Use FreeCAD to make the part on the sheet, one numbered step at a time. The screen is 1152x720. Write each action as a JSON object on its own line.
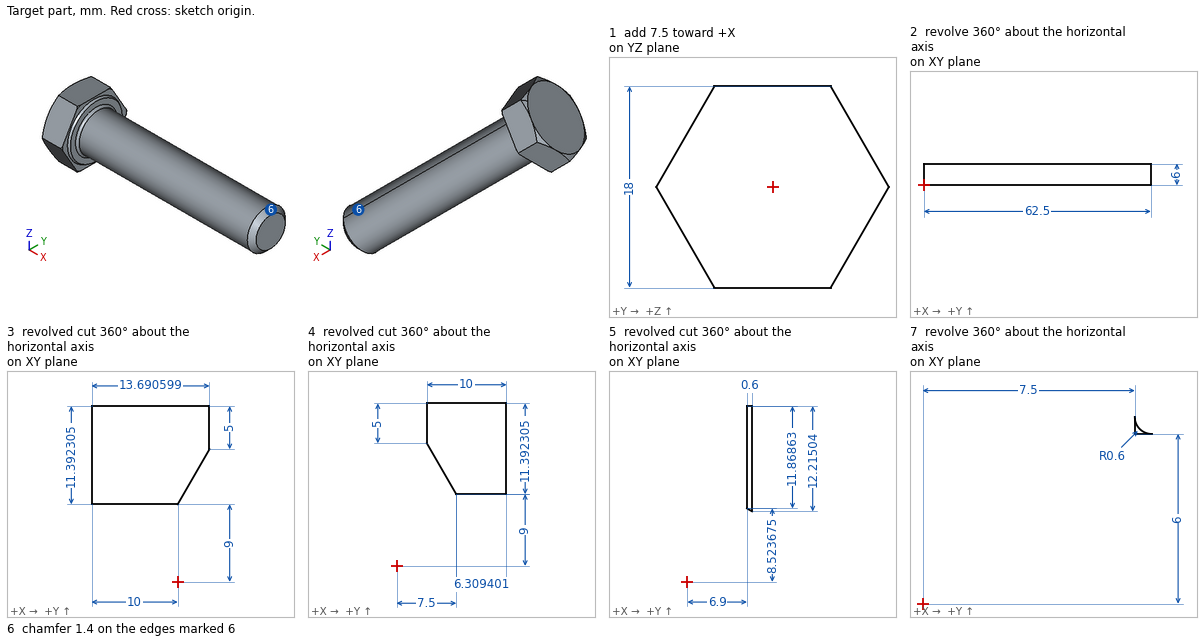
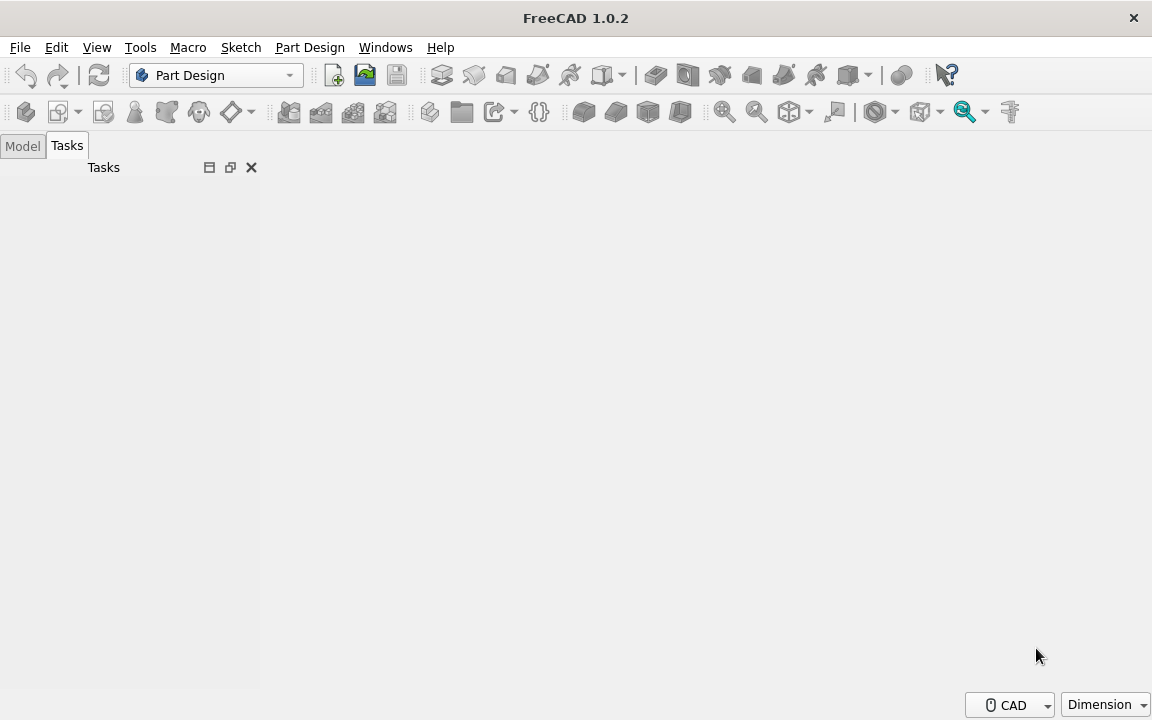
{"action": "key", "text": "ctrl+n"}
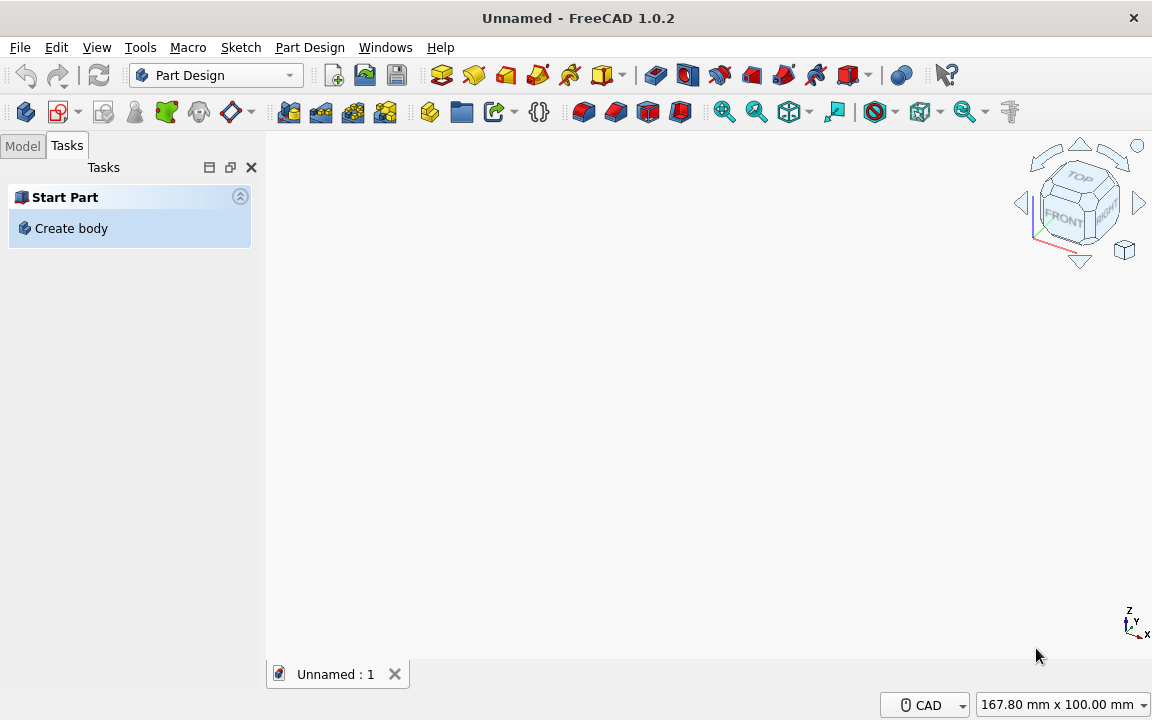
{"action": "left_click", "coordinate": [58, 112]}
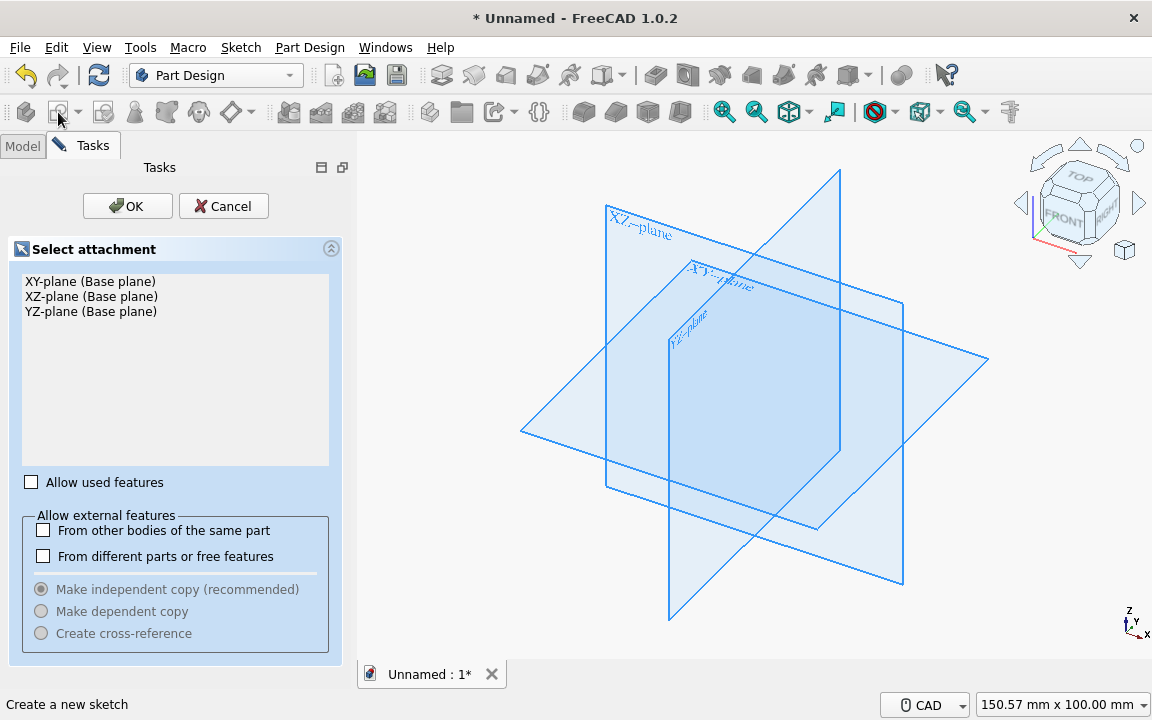
{"action": "left_click", "coordinate": [82, 312]}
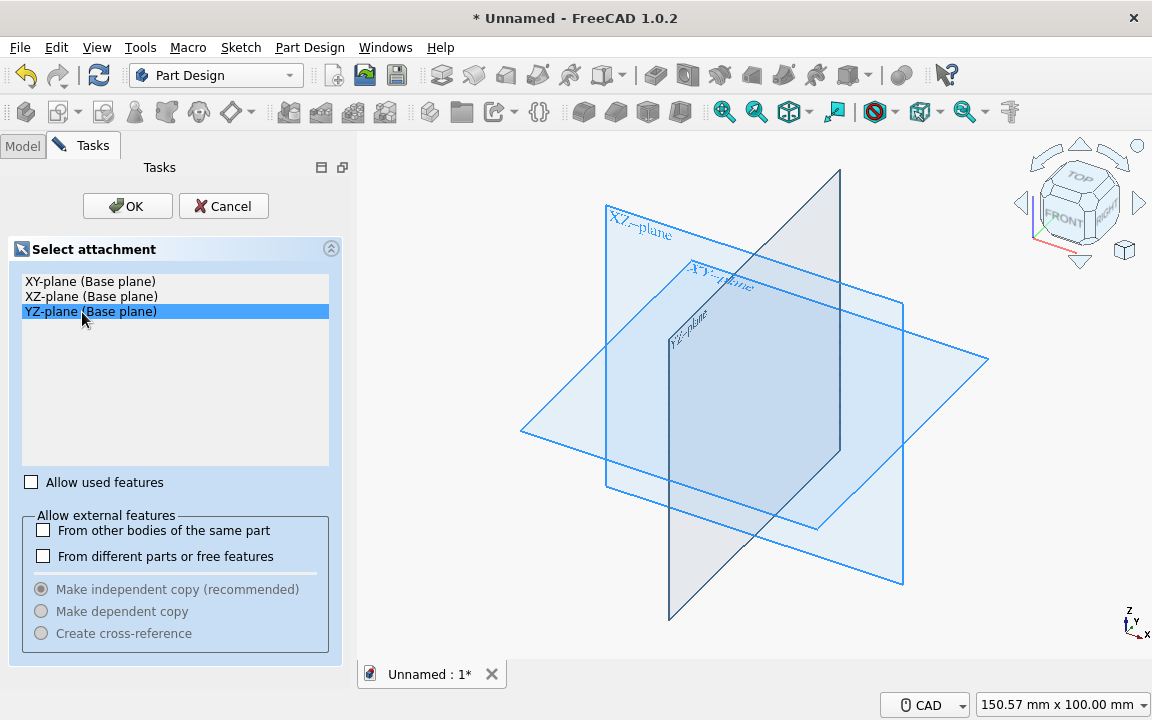
{"action": "left_click", "coordinate": [128, 206]}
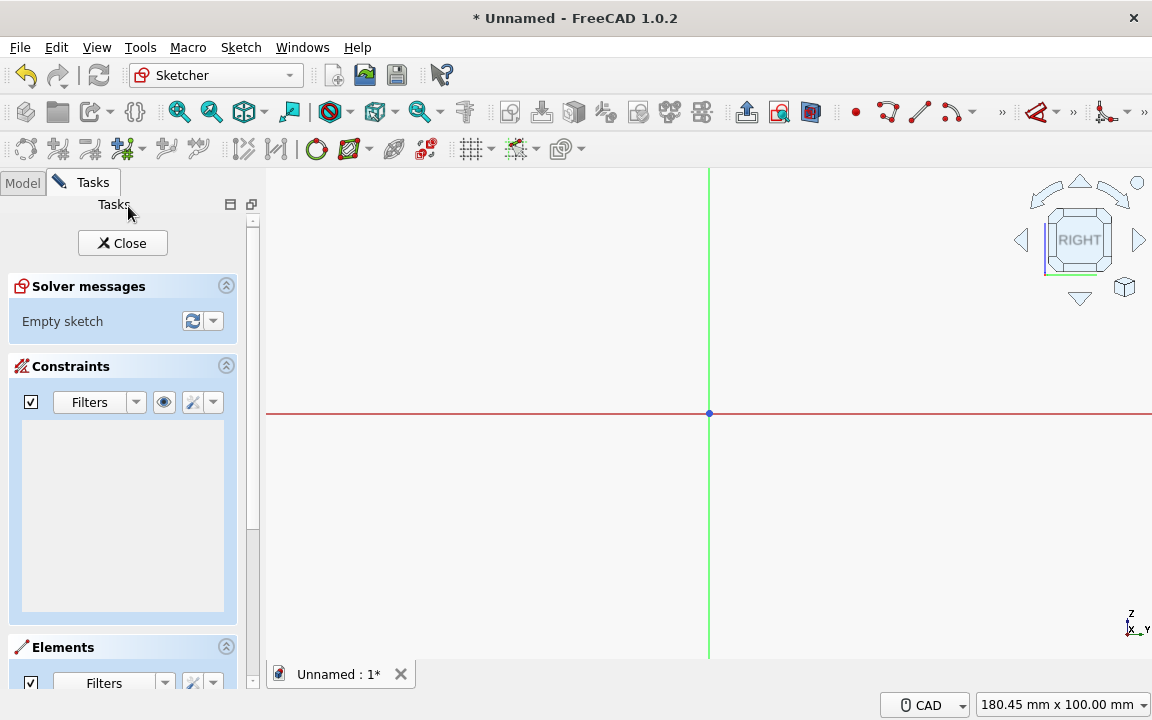
{"action": "scroll", "coordinate": [739, 414], "scroll_direction": "up", "scroll_amount": 6}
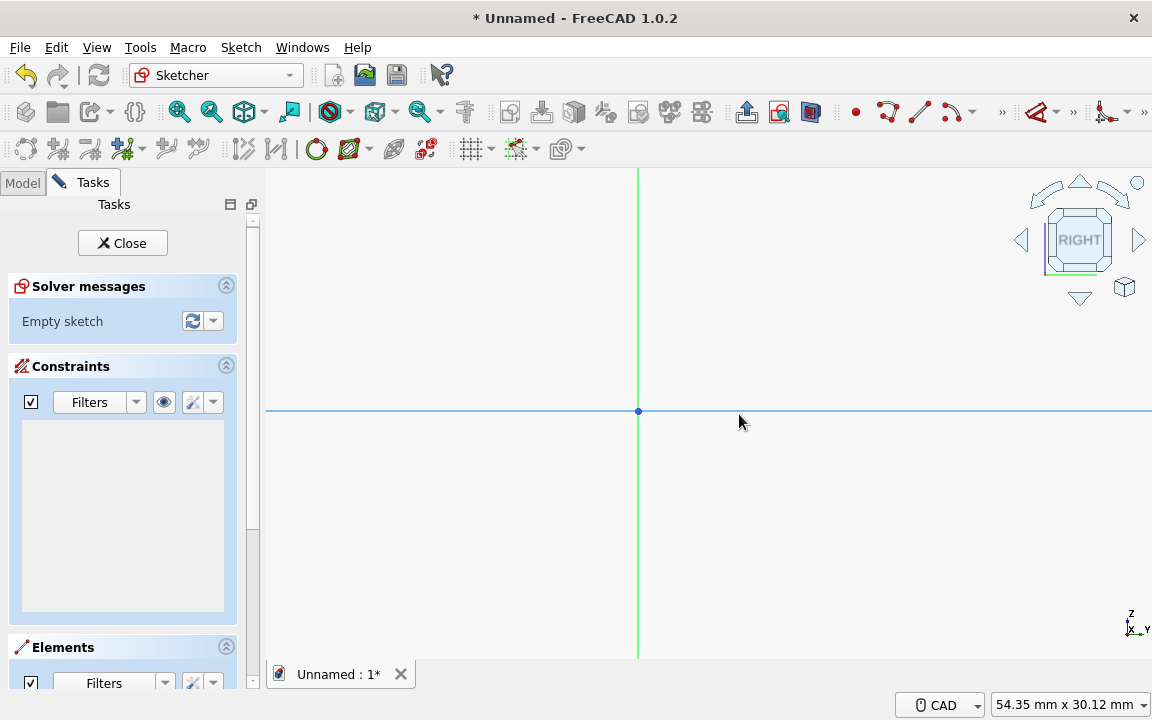
{"action": "key", "text": "g p 6"}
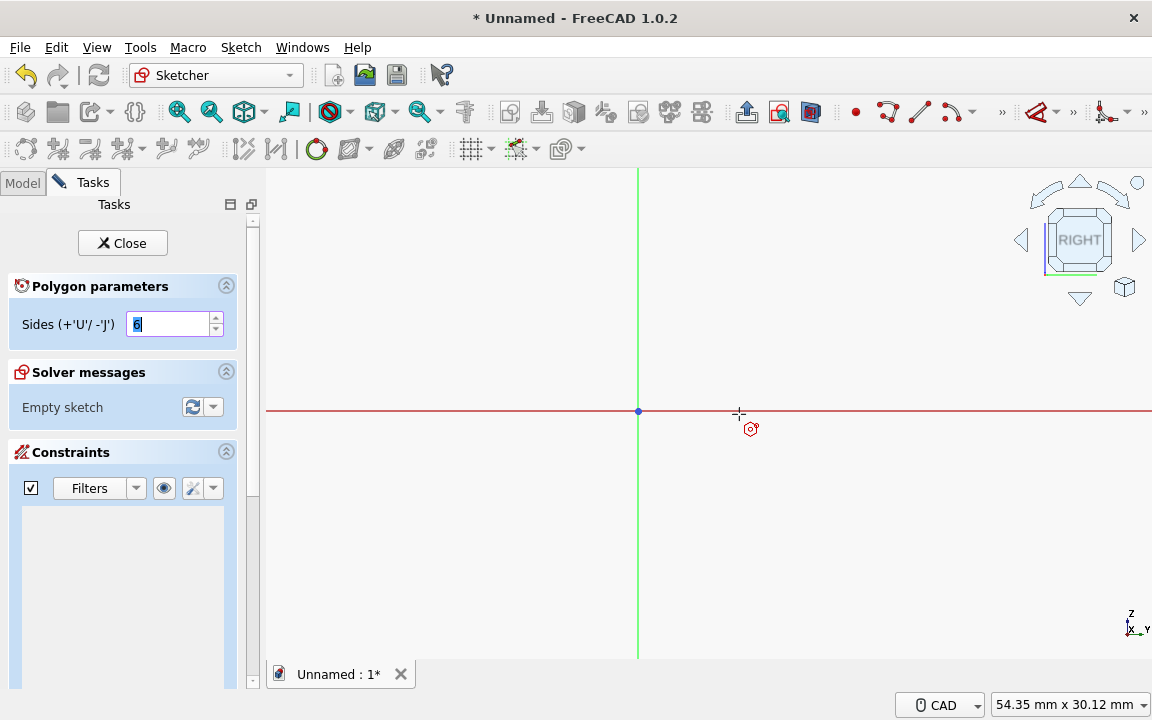
{"action": "left_click", "coordinate": [638, 411]}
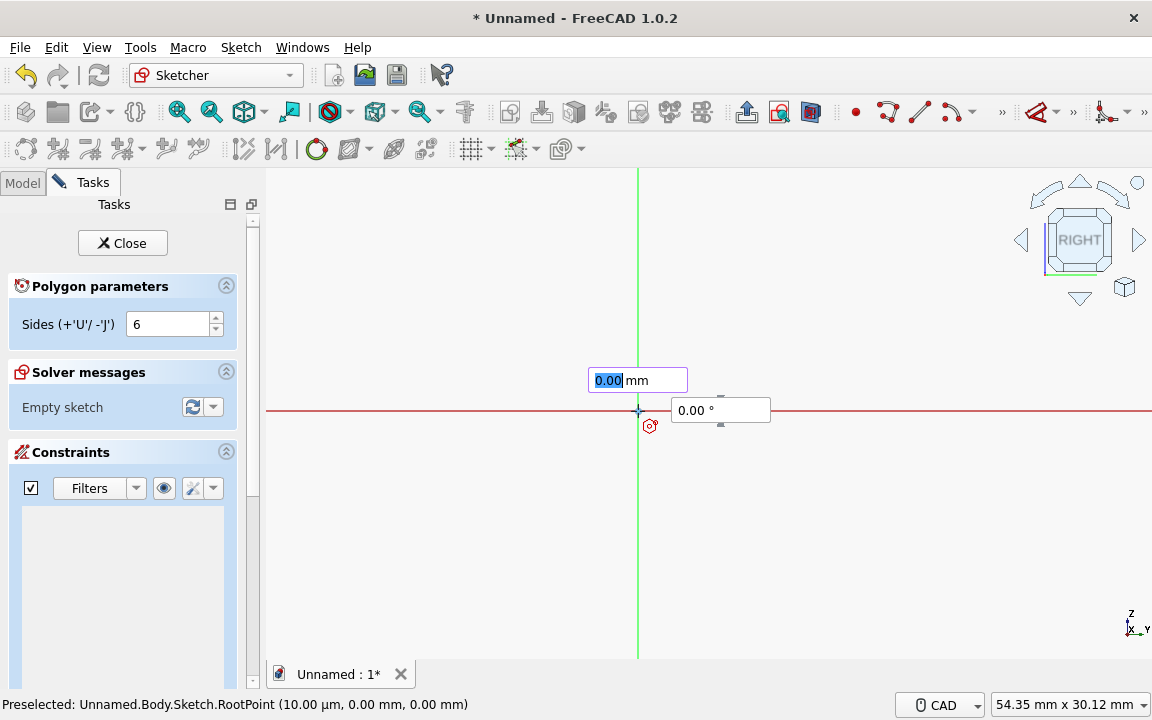
{"action": "left_click", "coordinate": [808, 411]}
{"action": "right_click", "coordinate": [808, 411]}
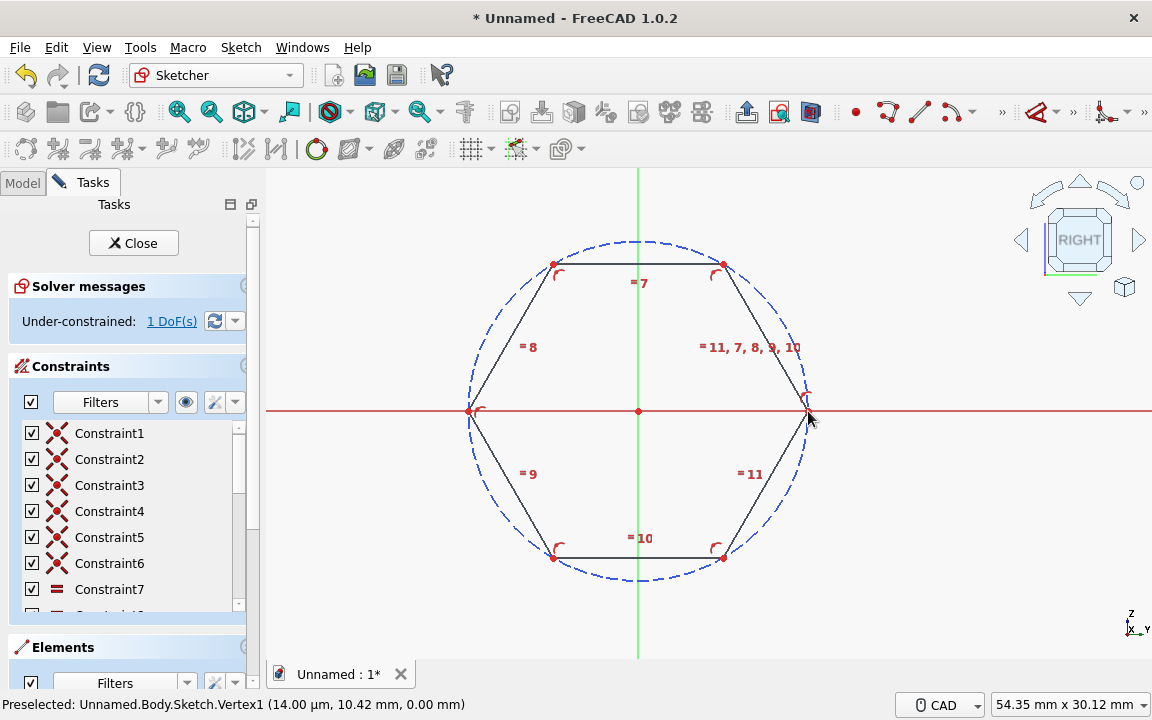
{"action": "key", "text": "d"}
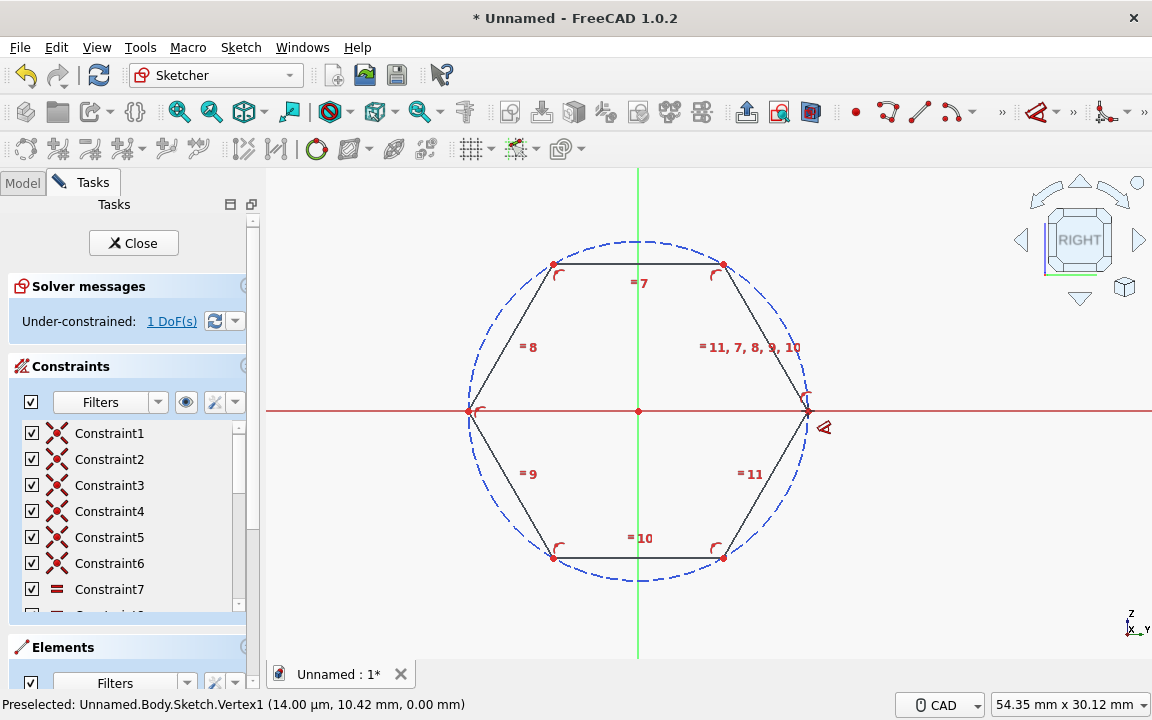
{"action": "left_click", "coordinate": [553, 558]}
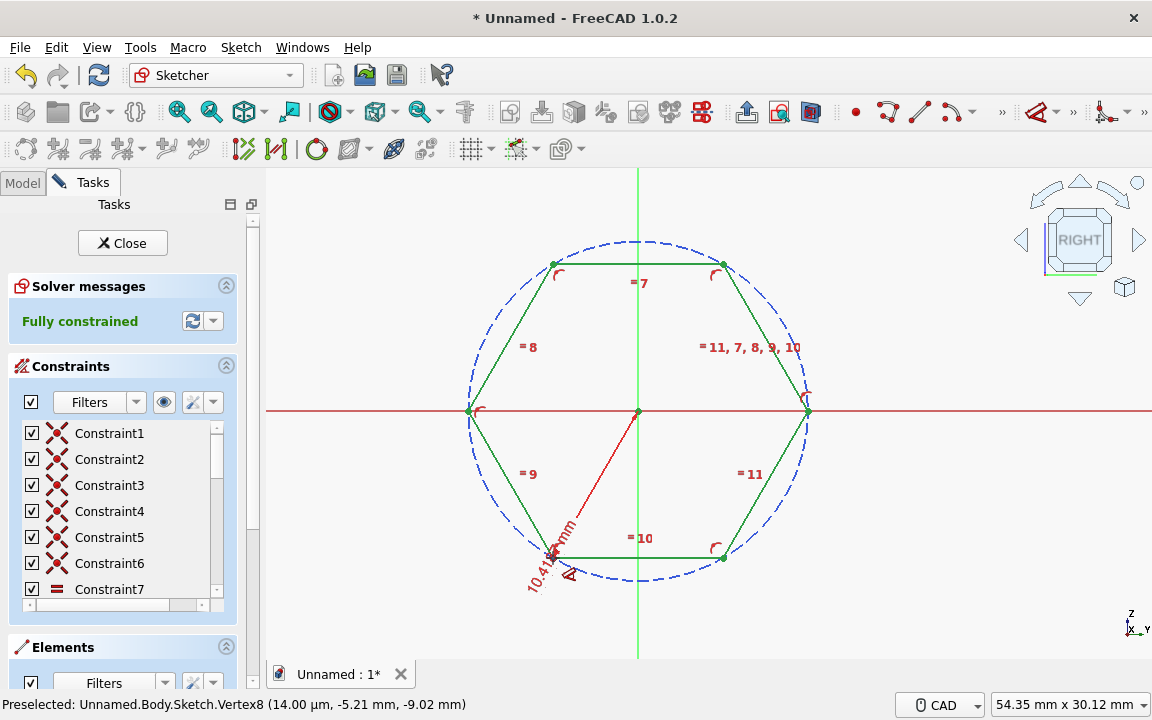
{"action": "left_click", "coordinate": [723, 264]}
{"action": "left_click", "coordinate": [471, 308]}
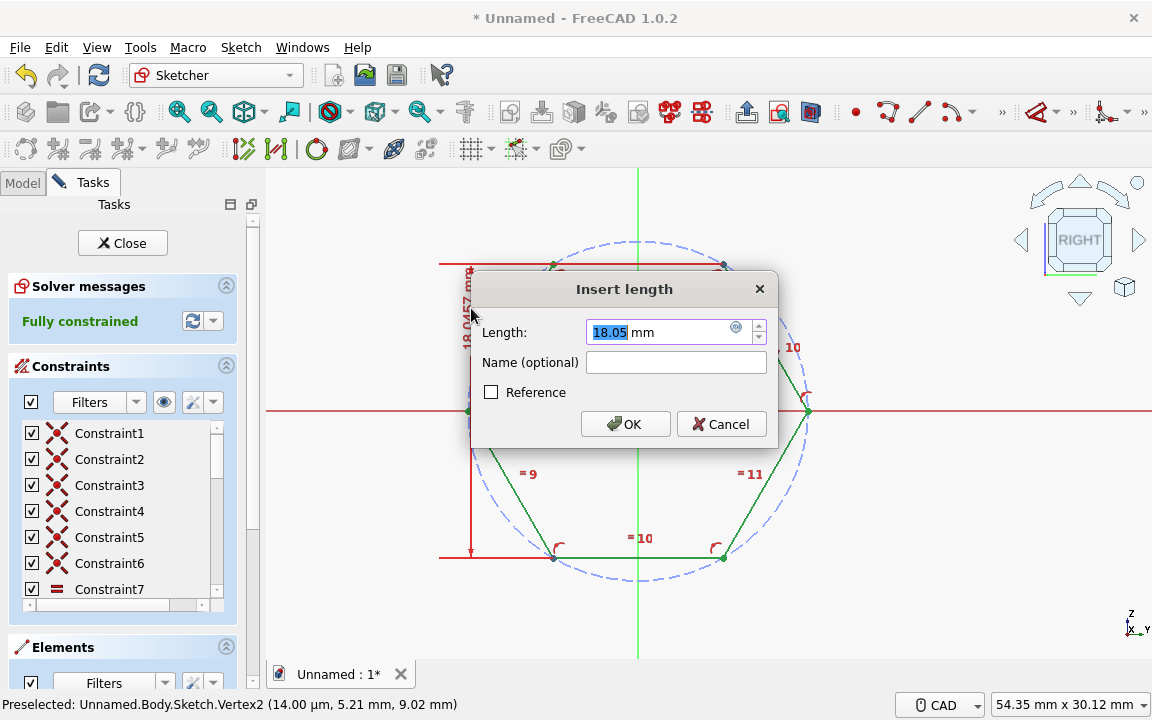
{"action": "type", "text": "18"}
{"action": "key", "text": "Return"}
{"action": "key", "text": "Escape"}